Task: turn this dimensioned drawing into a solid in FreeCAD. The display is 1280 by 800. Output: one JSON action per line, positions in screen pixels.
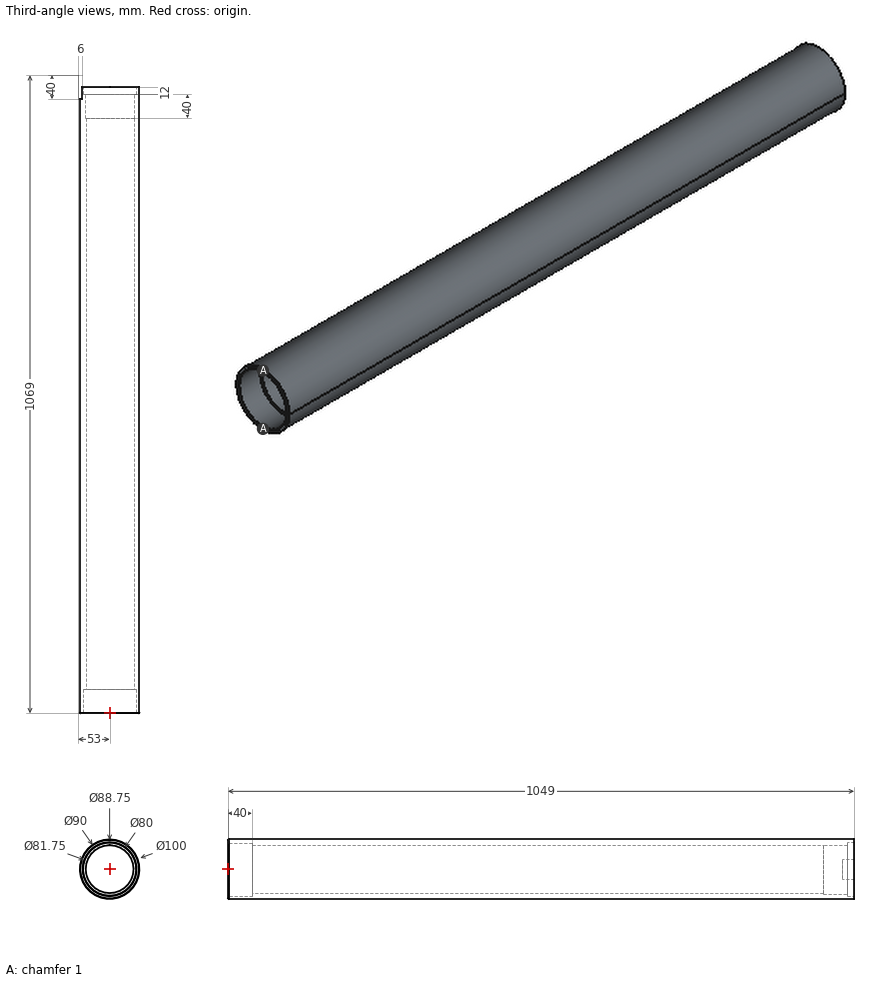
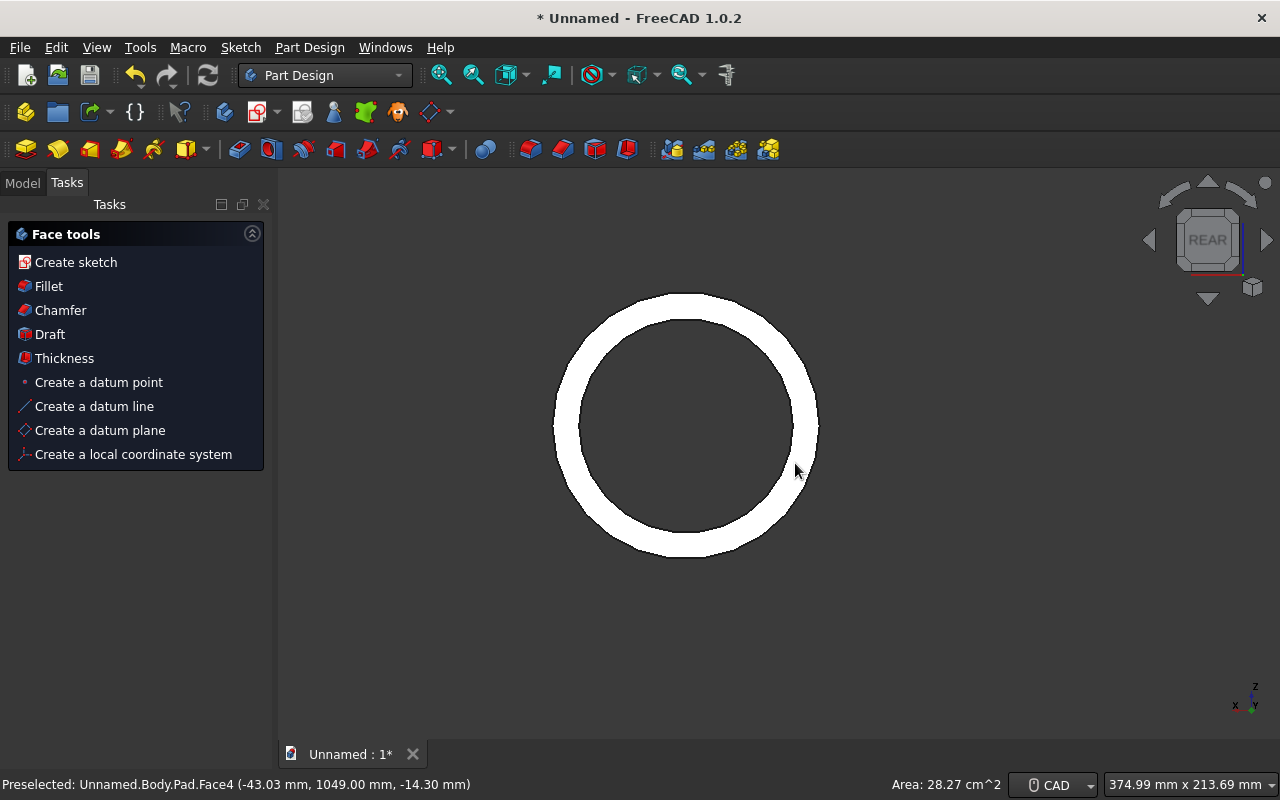
{"action": "left_click", "coordinate": [258, 112]}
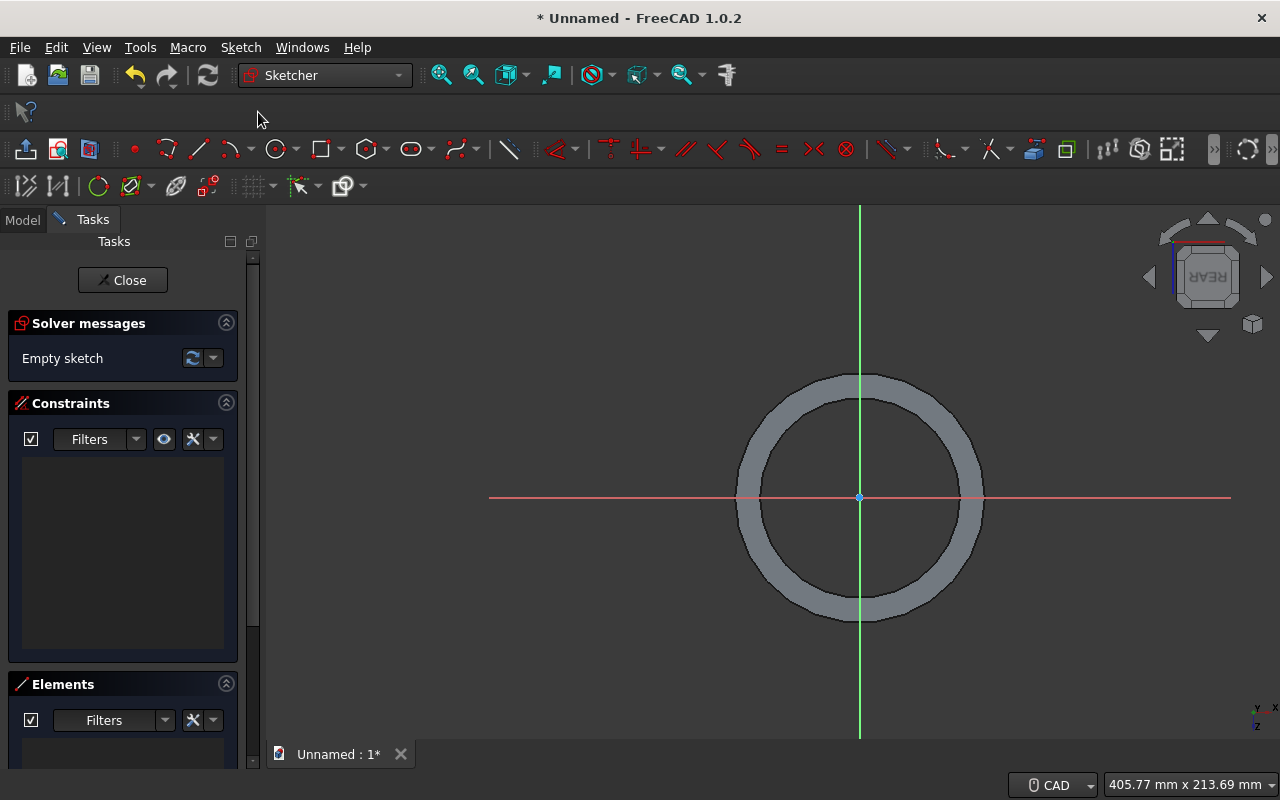
{"action": "scroll", "coordinate": [1115, 551], "scroll_direction": "up", "scroll_amount": 2}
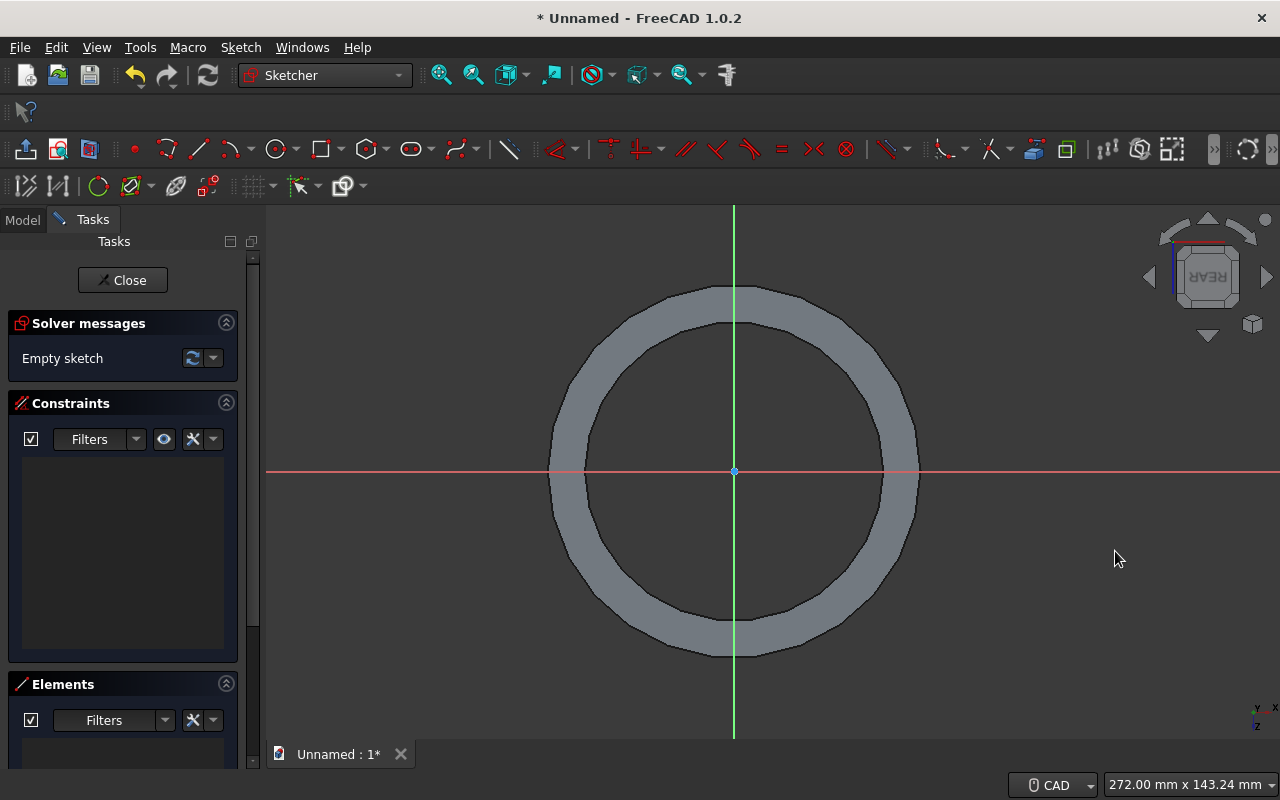
{"action": "left_click", "coordinate": [276, 150]}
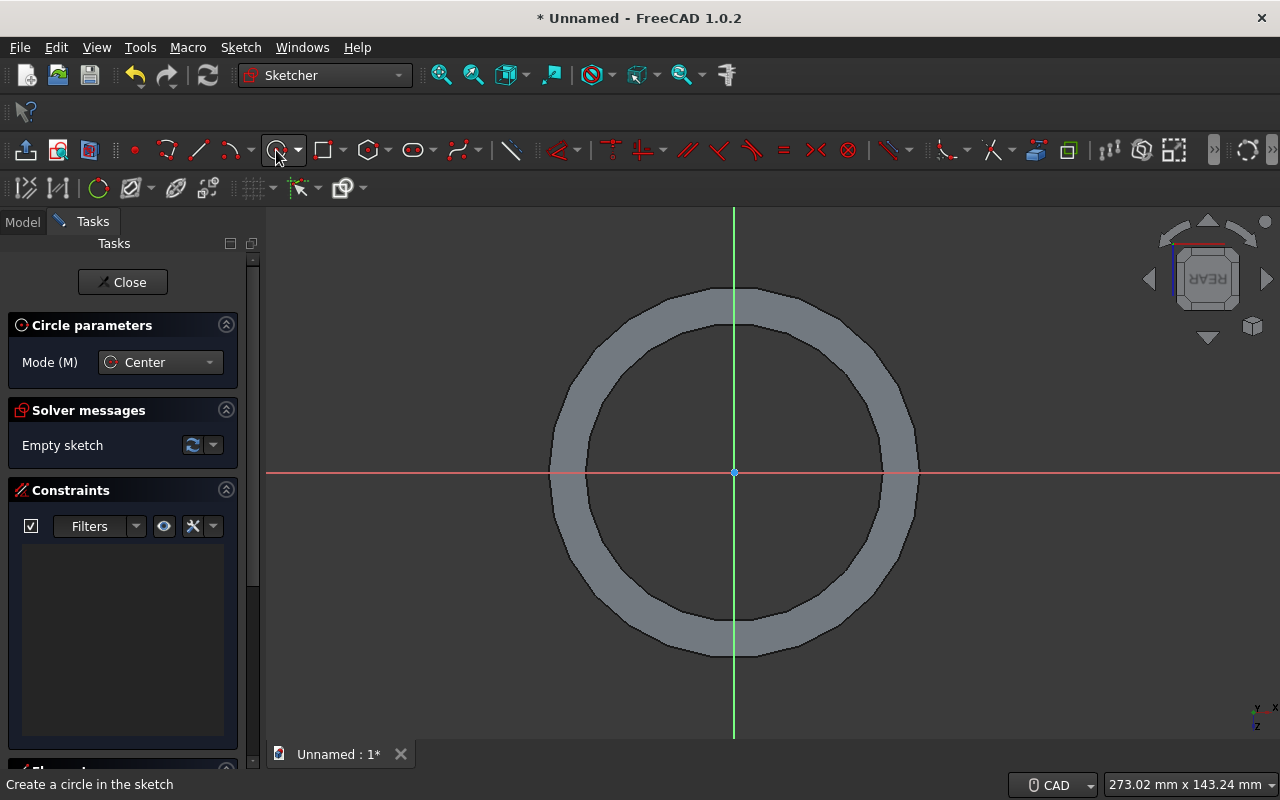
{"action": "left_click", "coordinate": [734, 473]}
{"action": "mouse_move", "coordinate": [852, 354]}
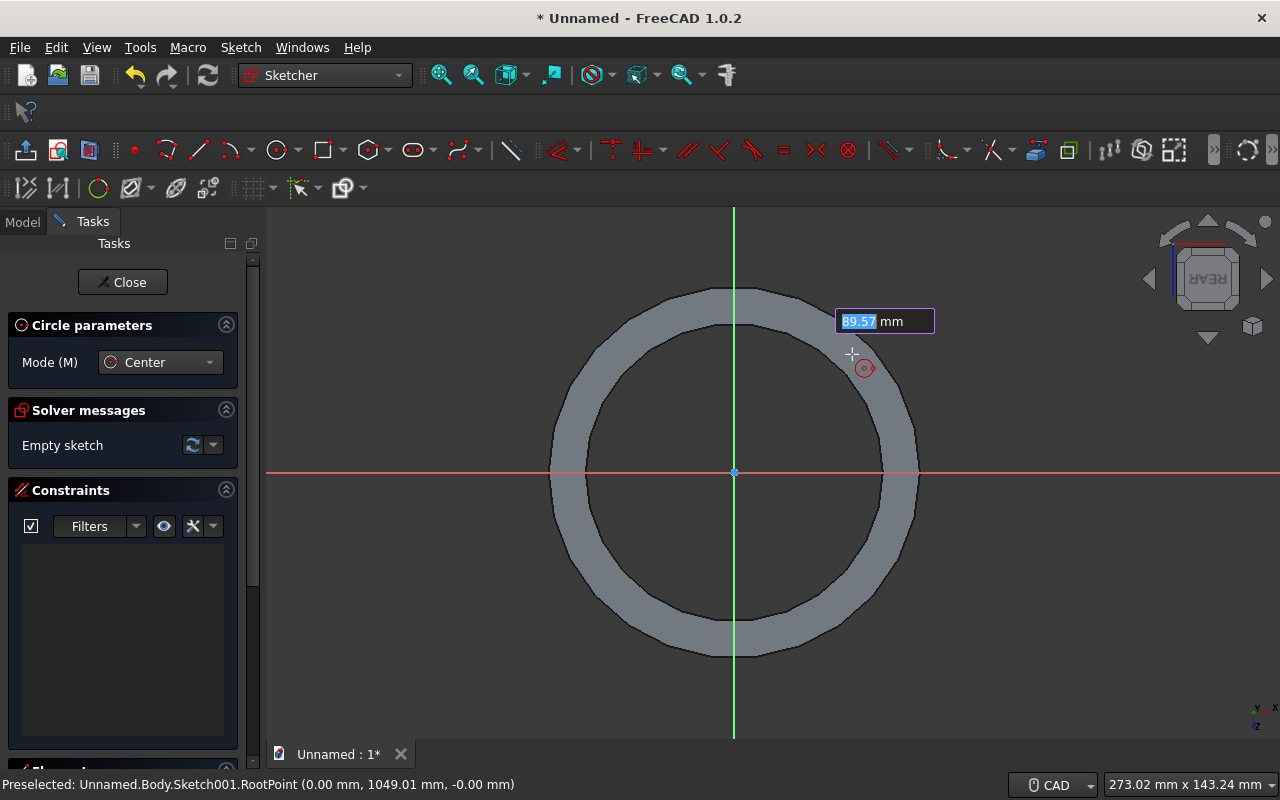
{"action": "type", "text": "90"}
{"action": "key", "text": "Return"}
{"action": "key", "text": "Escape"}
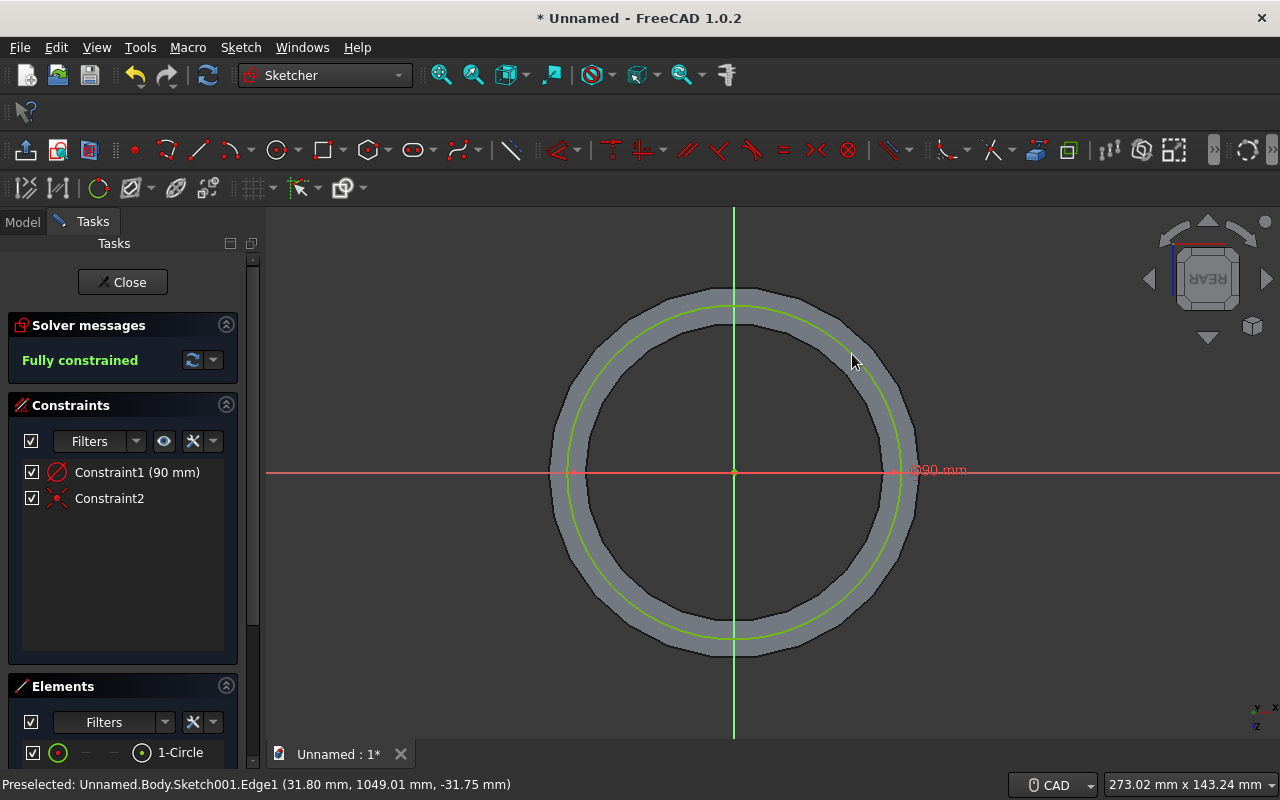
{"action": "left_click", "coordinate": [123, 282]}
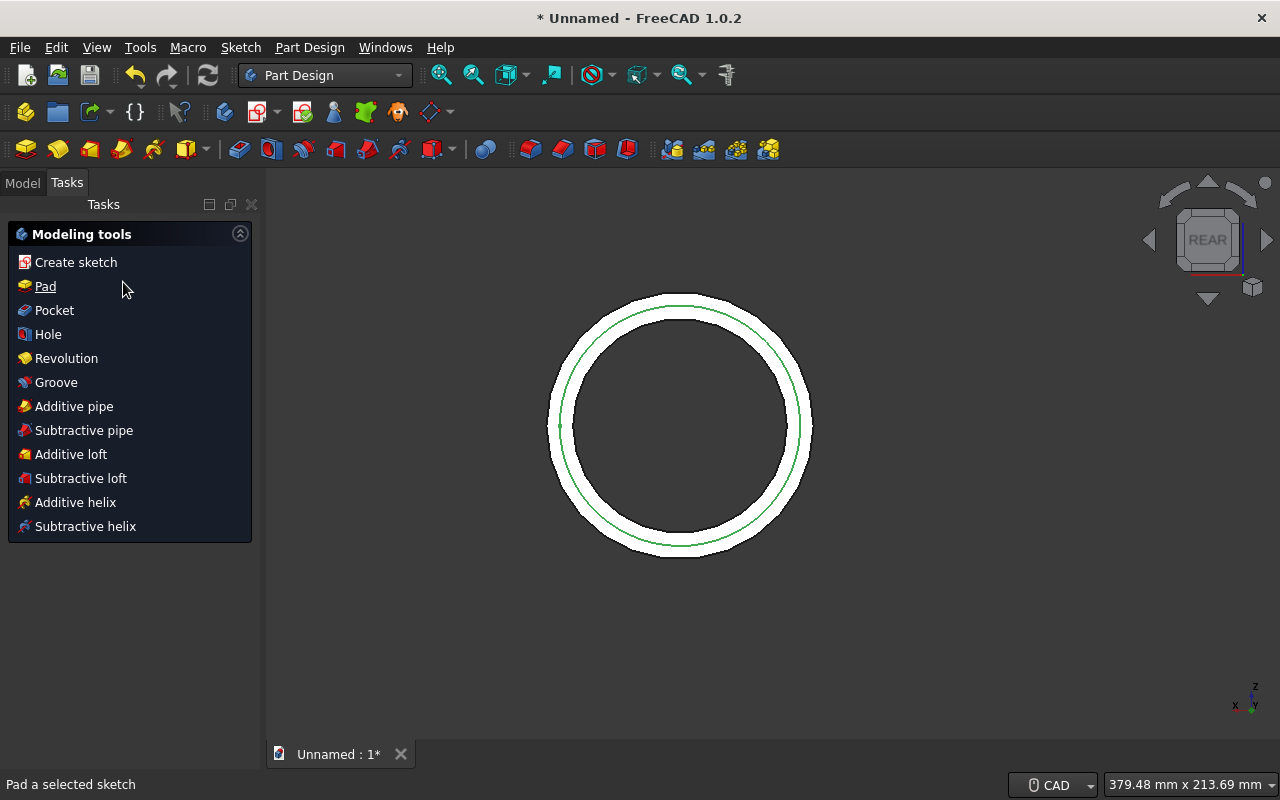
{"action": "left_click", "coordinate": [240, 150]}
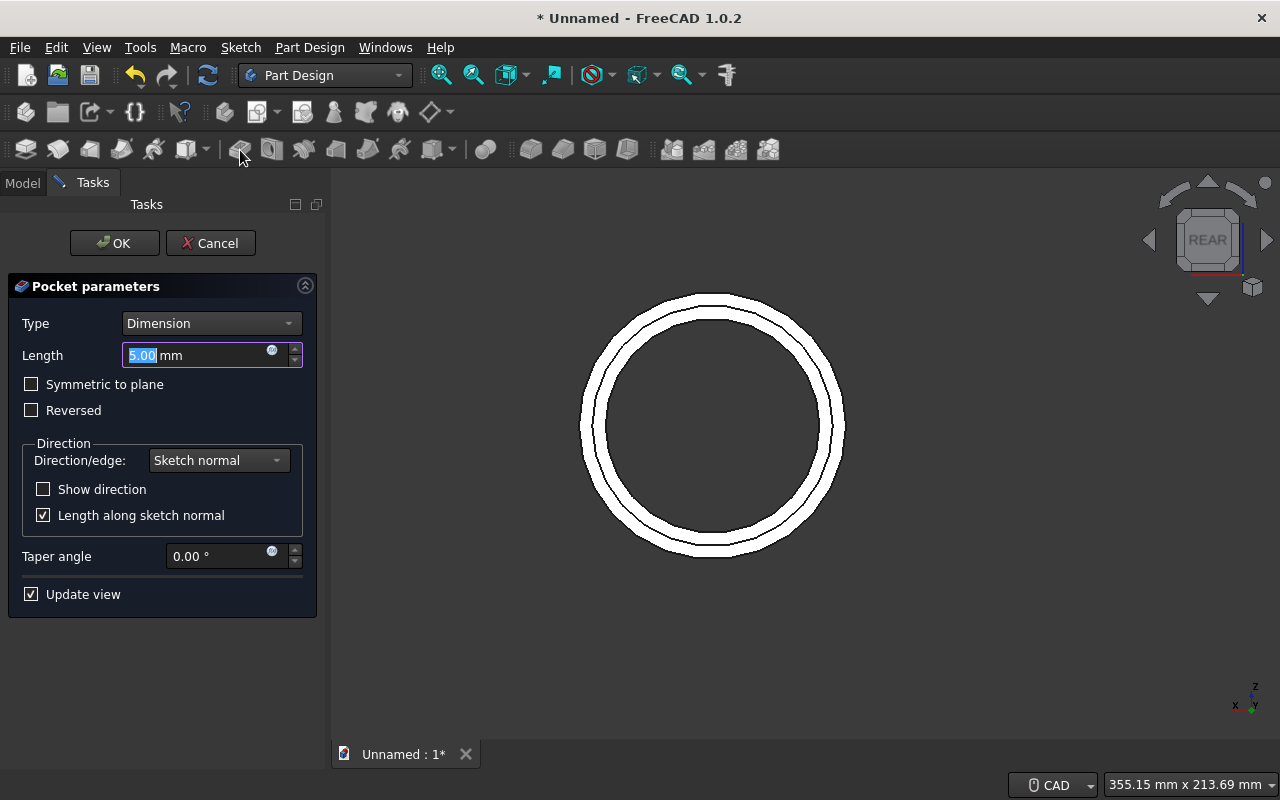
{"action": "type", "text": "12"}
{"action": "key", "text": "Tab"}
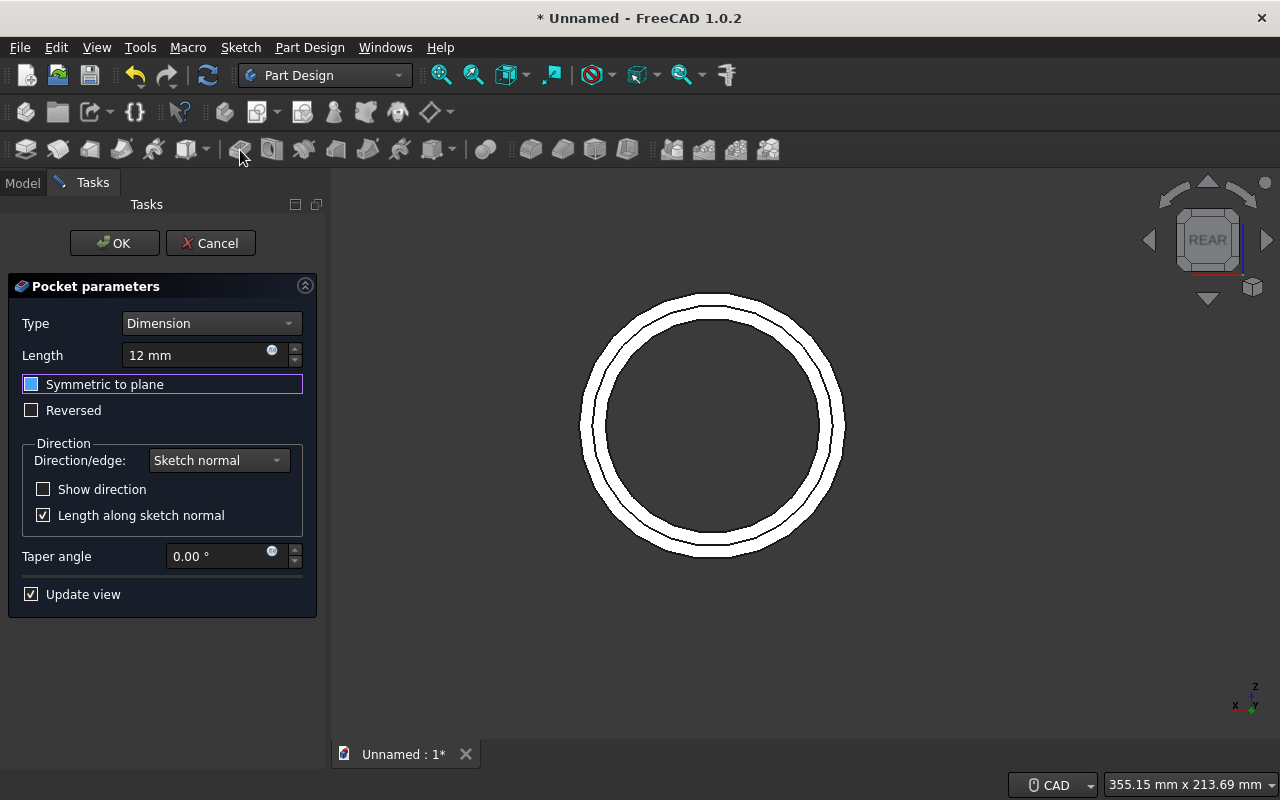
{"action": "left_click", "coordinate": [115, 243]}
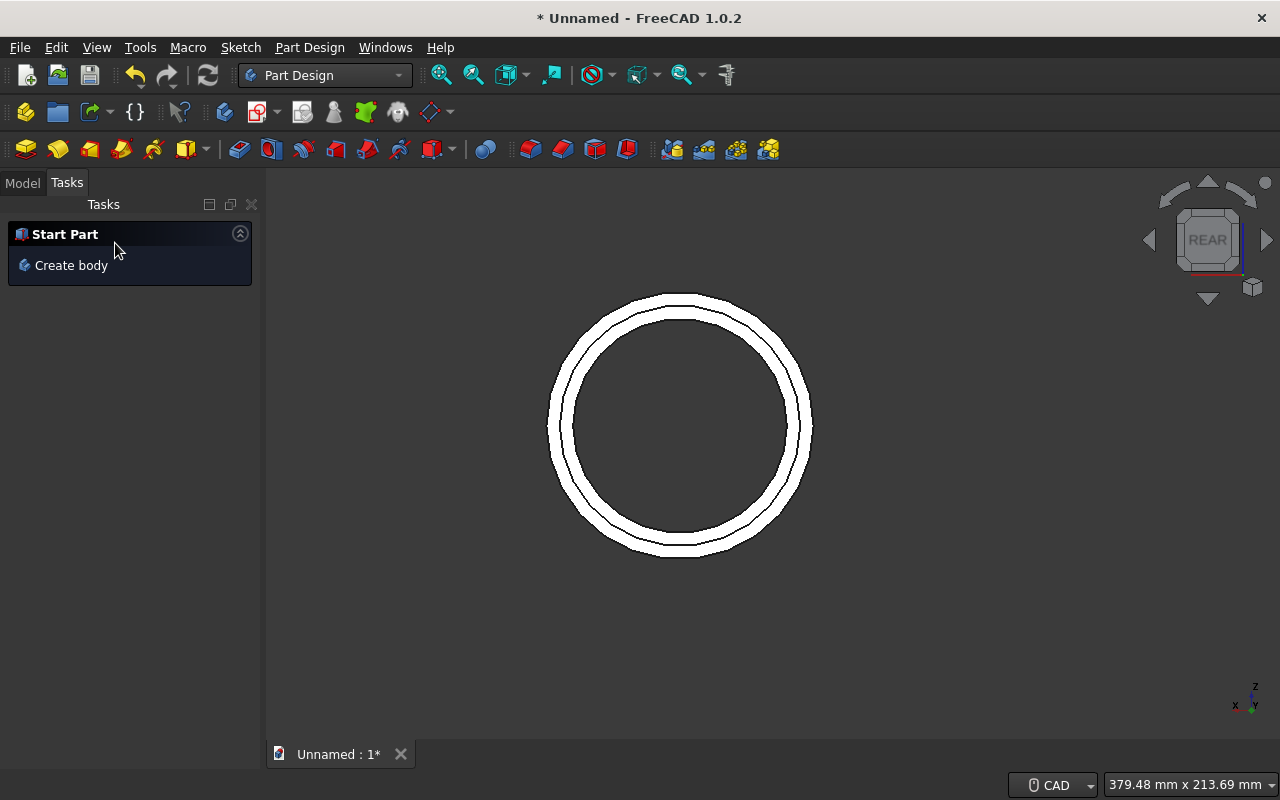
{"action": "key", "text": "0"}